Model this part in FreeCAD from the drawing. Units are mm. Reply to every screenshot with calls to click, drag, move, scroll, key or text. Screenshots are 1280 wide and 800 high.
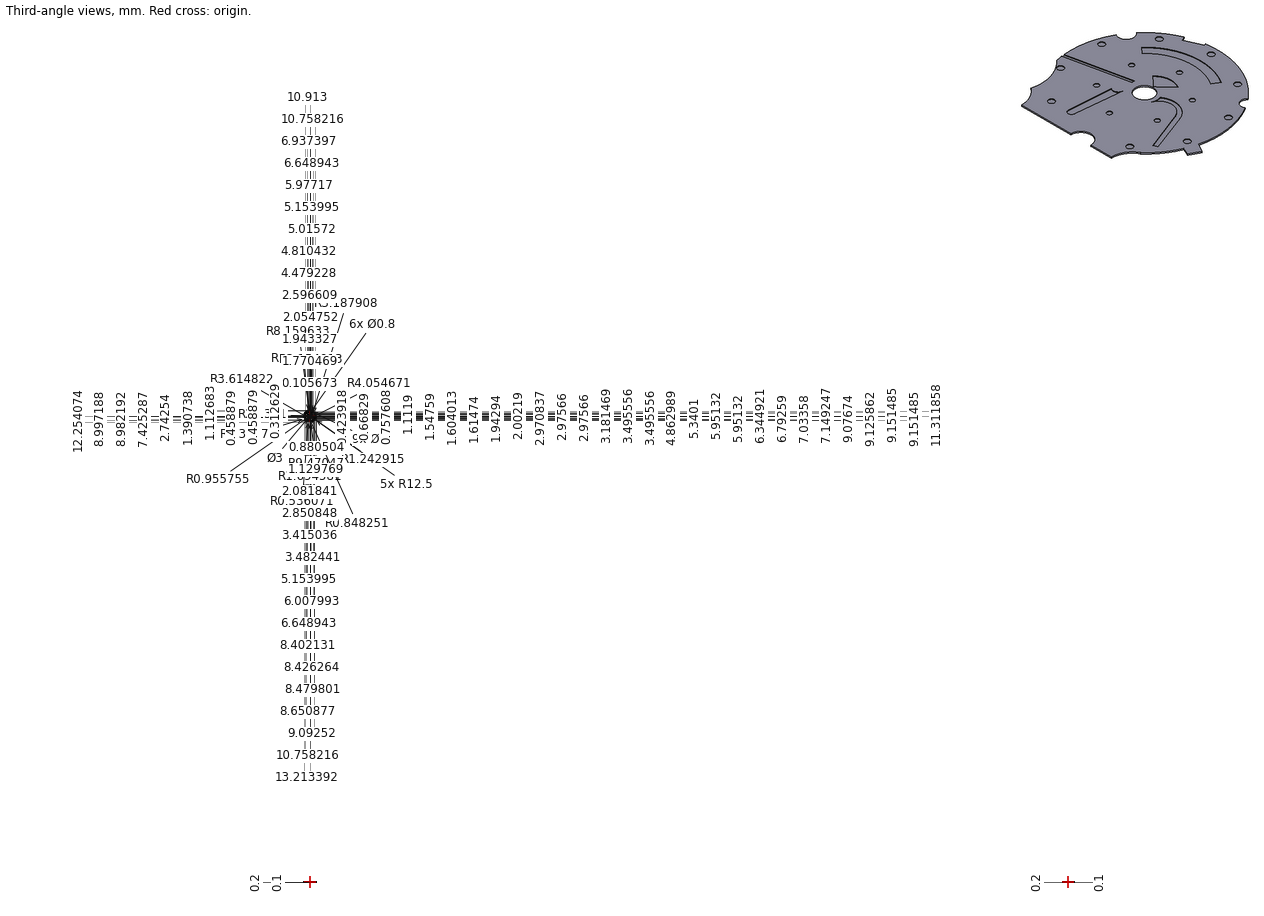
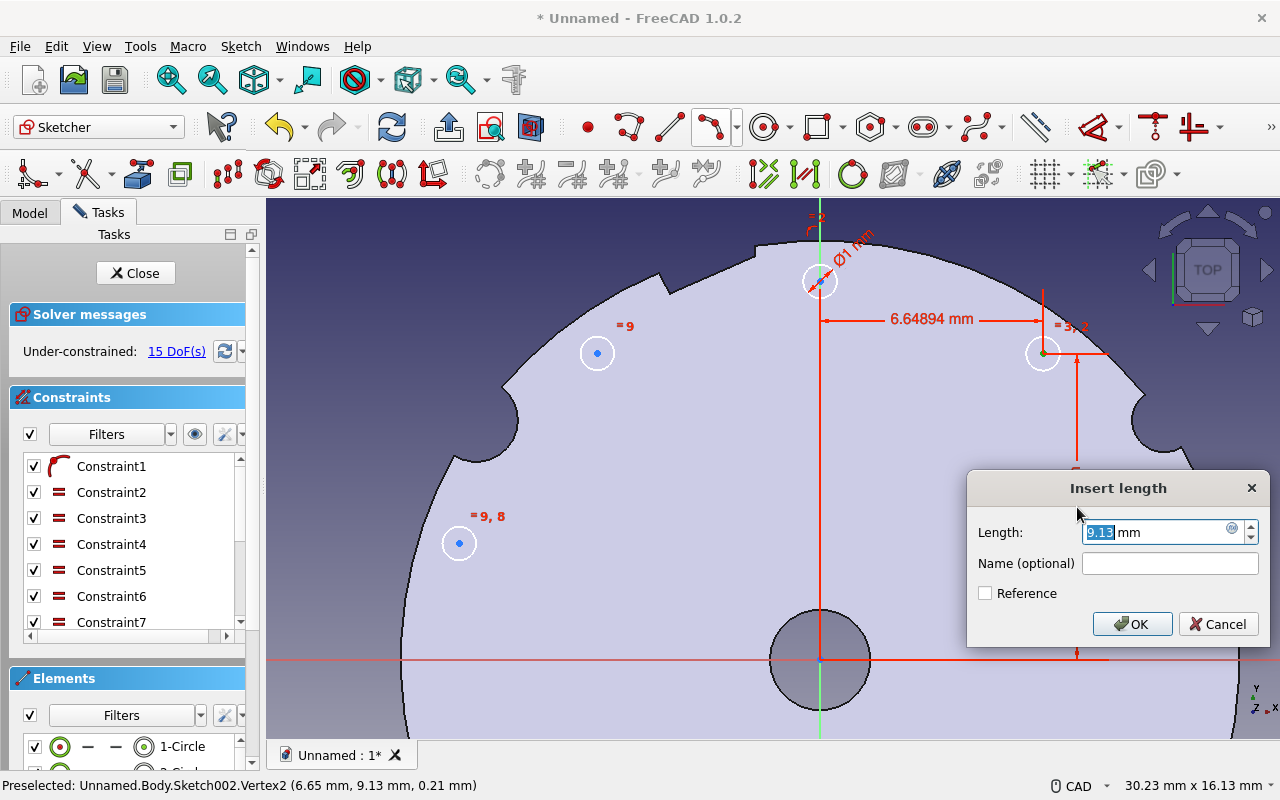
text(9.151485)
key(Return)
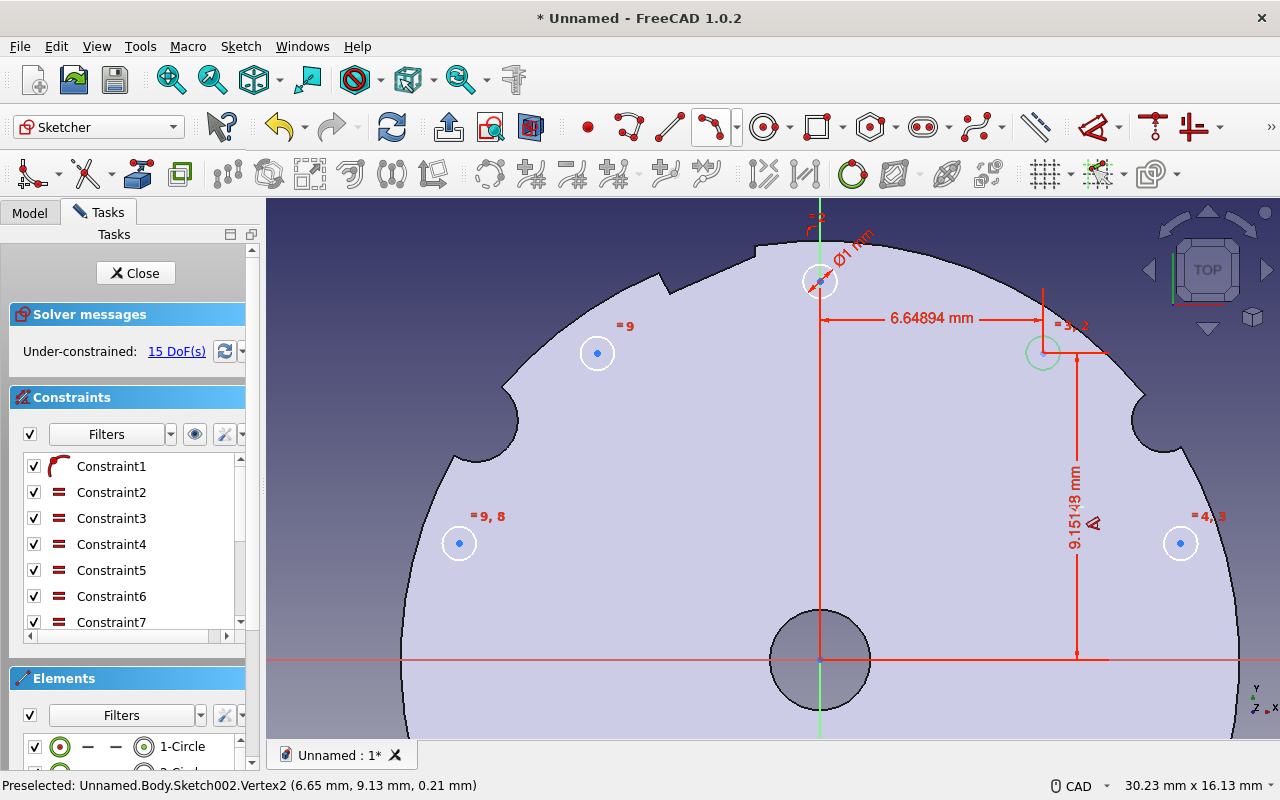
scroll(610, 342, down, 4)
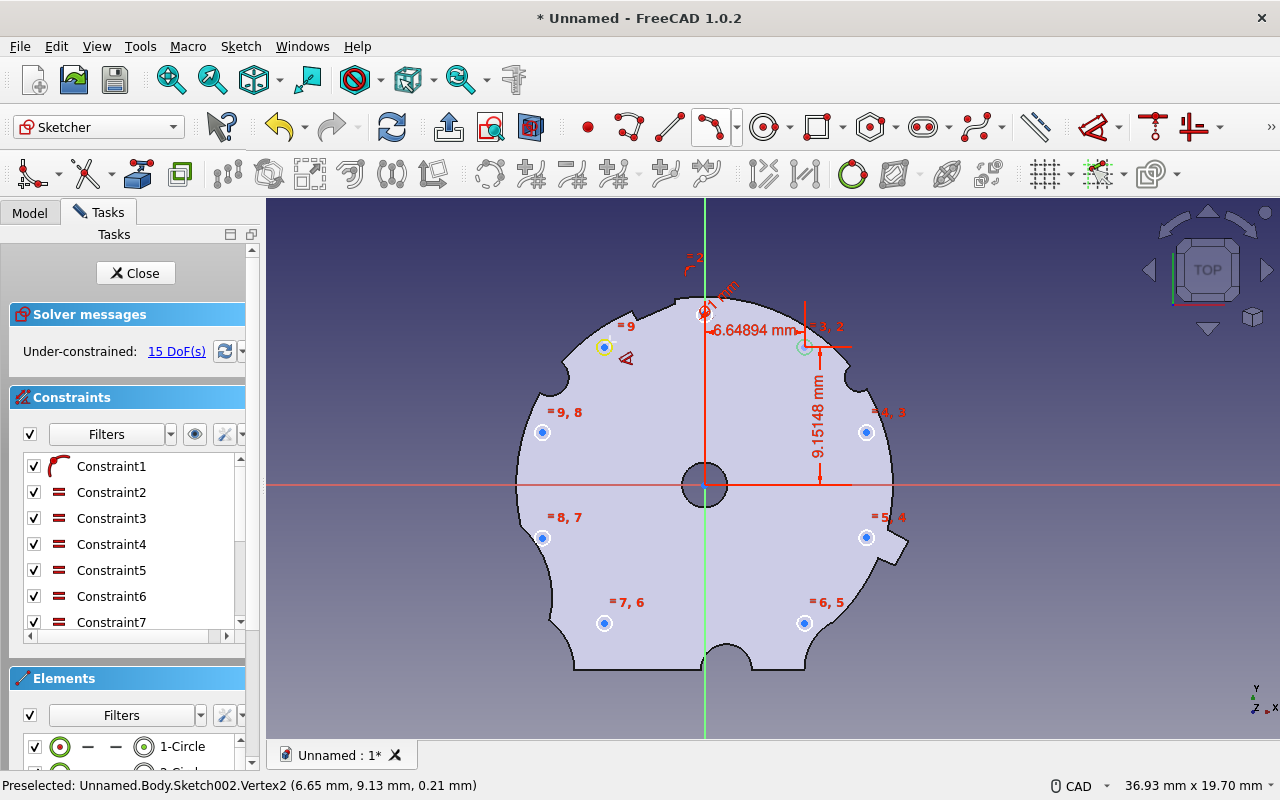
click(867, 433)
click(901, 459)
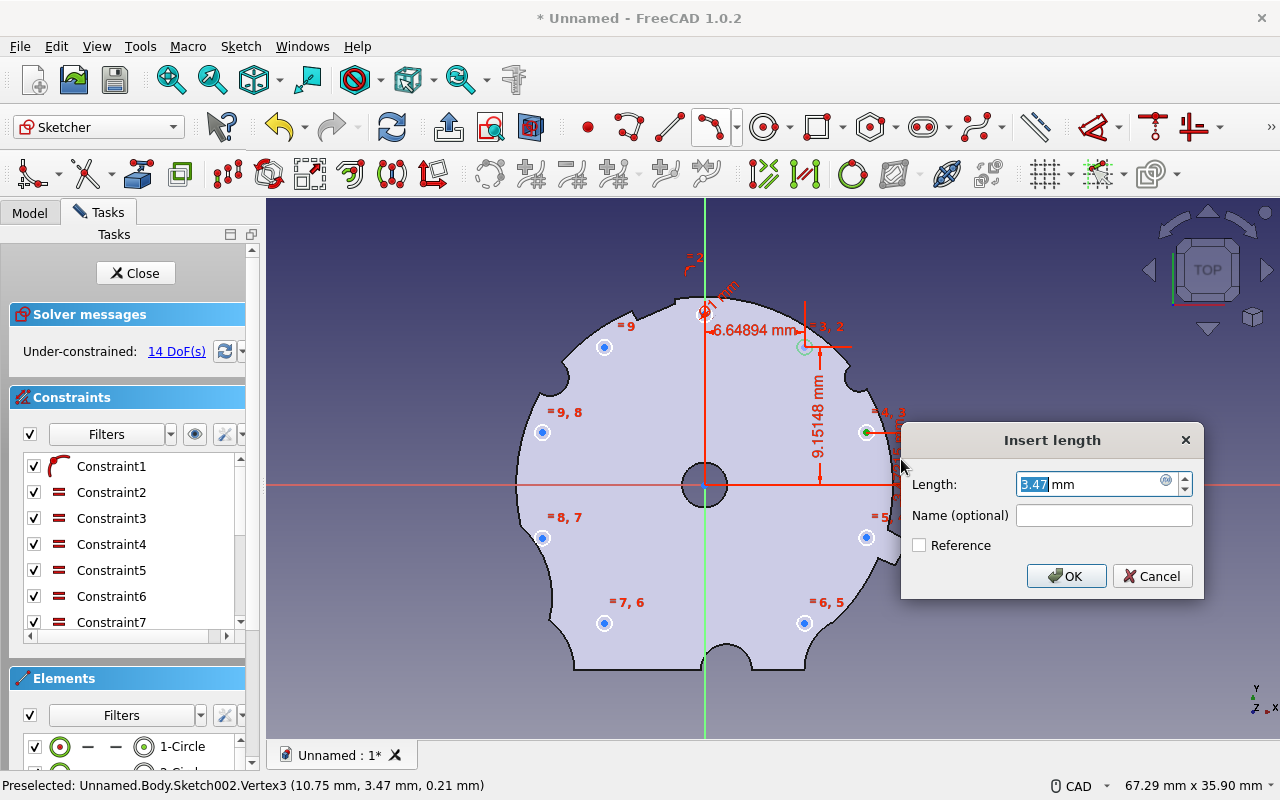
text(3.495556)
key(Return)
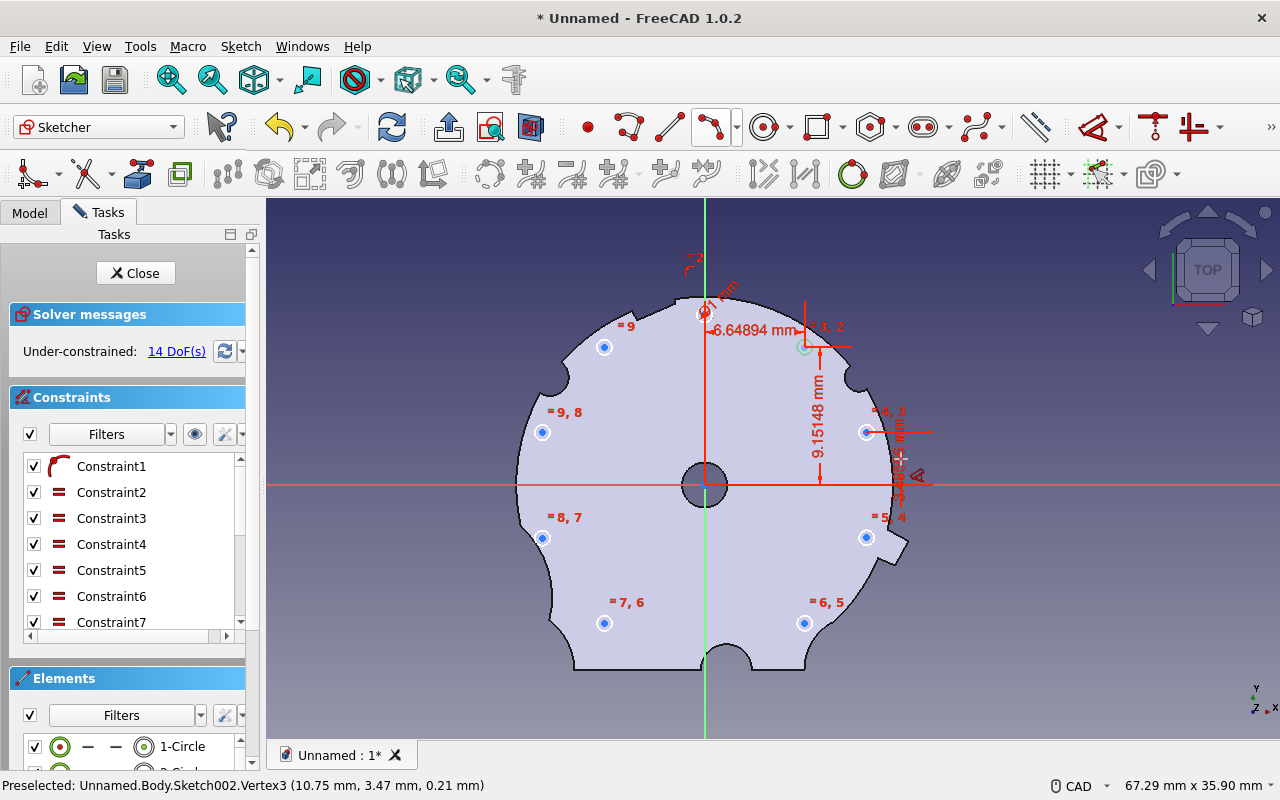
click(867, 538)
click(901, 511)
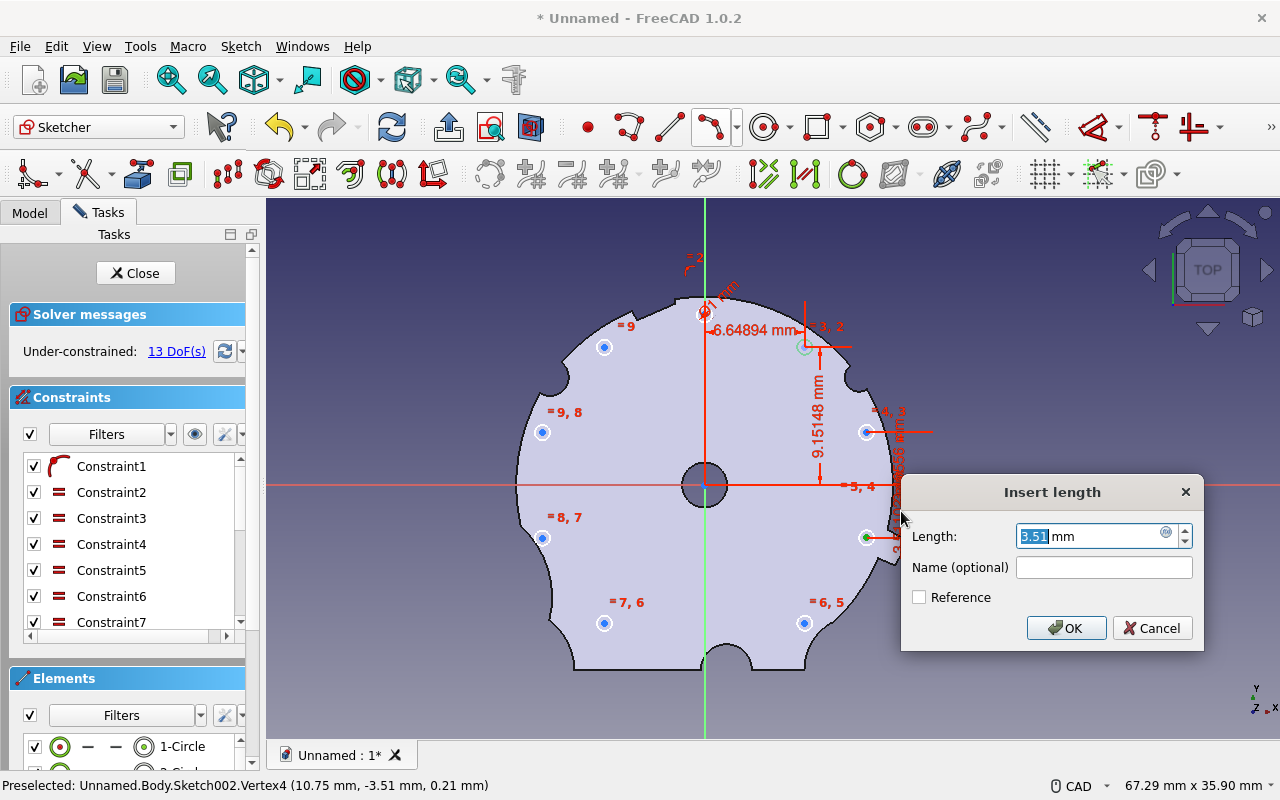
text(3.495556)
key(Return)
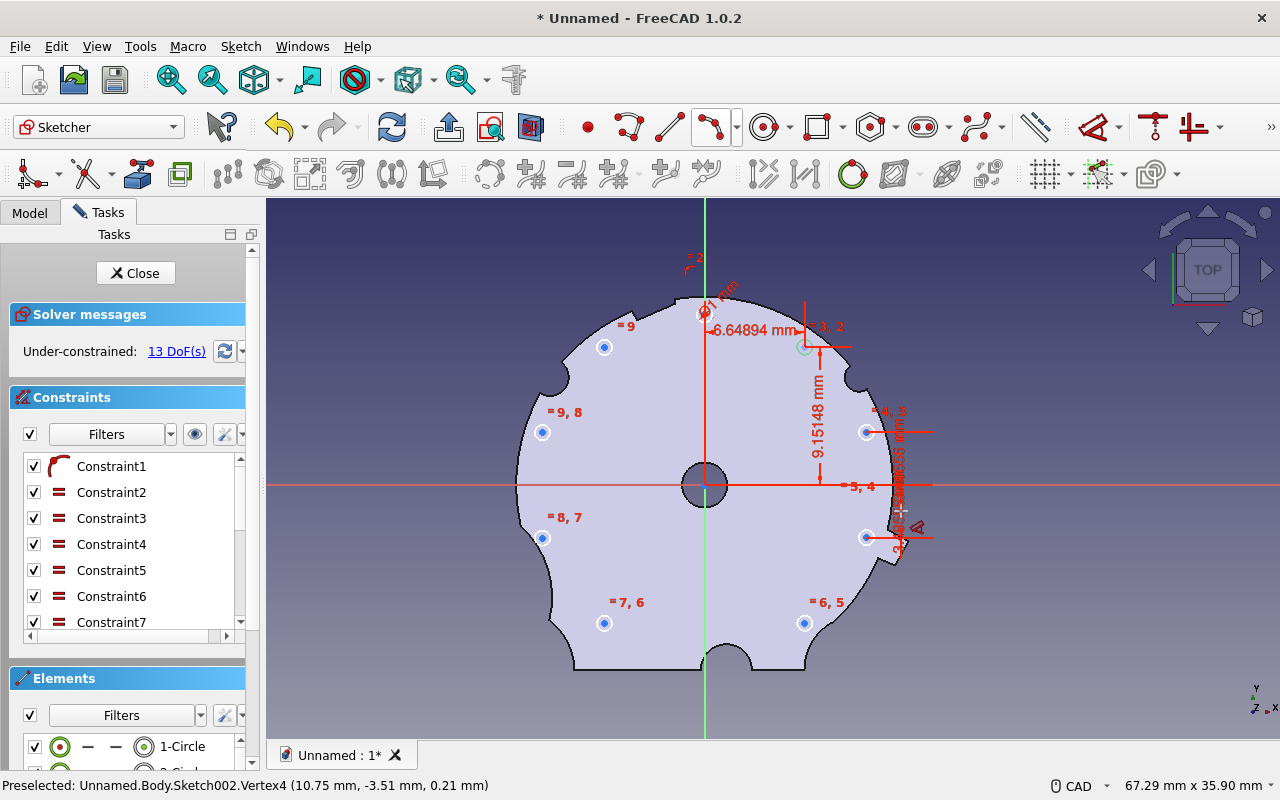
click(805, 623)
click(755, 657)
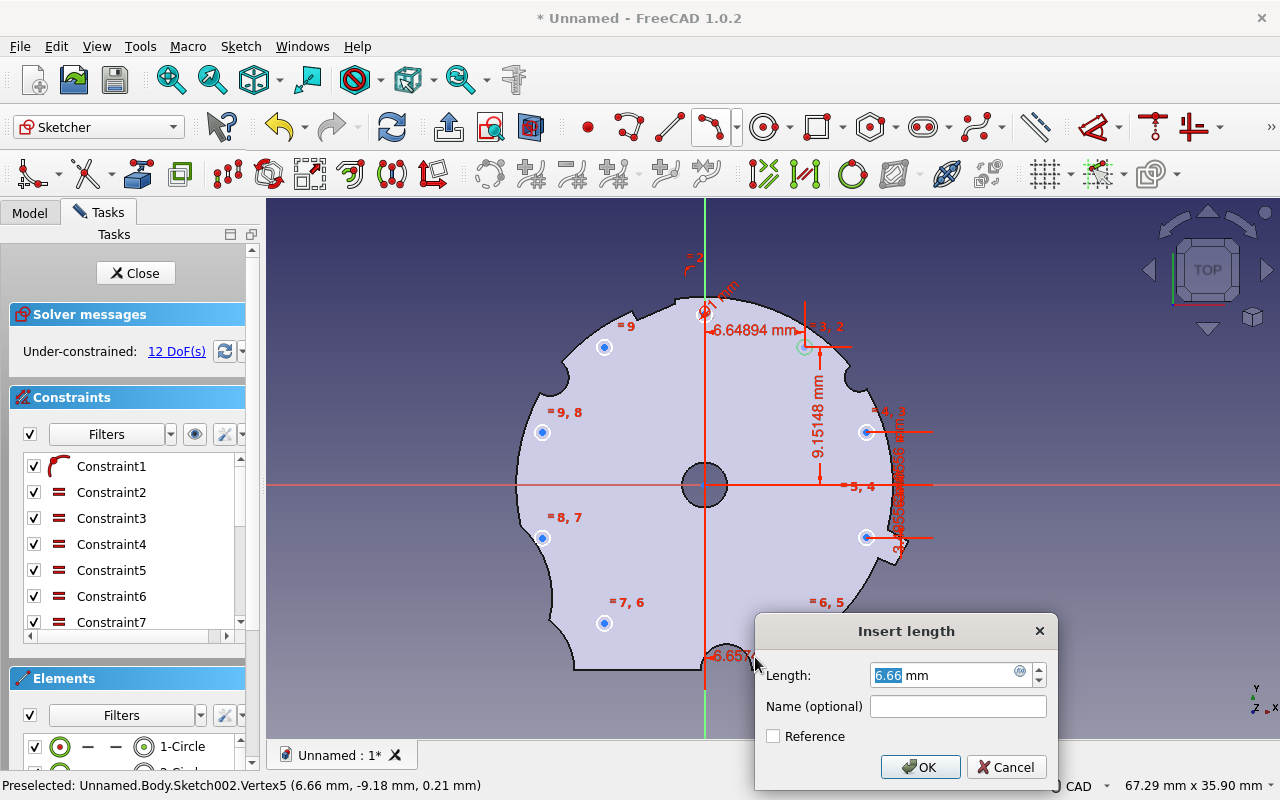
text(6.648943)
key(Return)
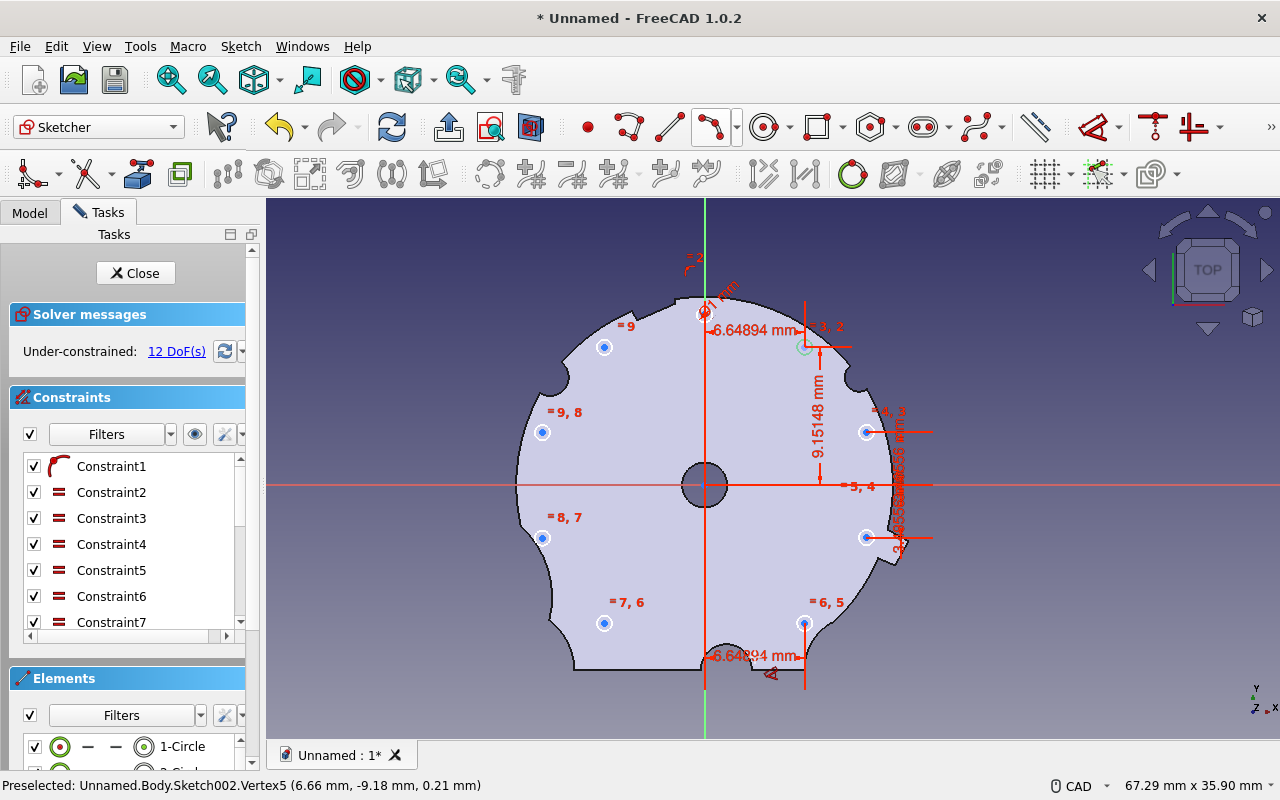
click(805, 623)
click(839, 554)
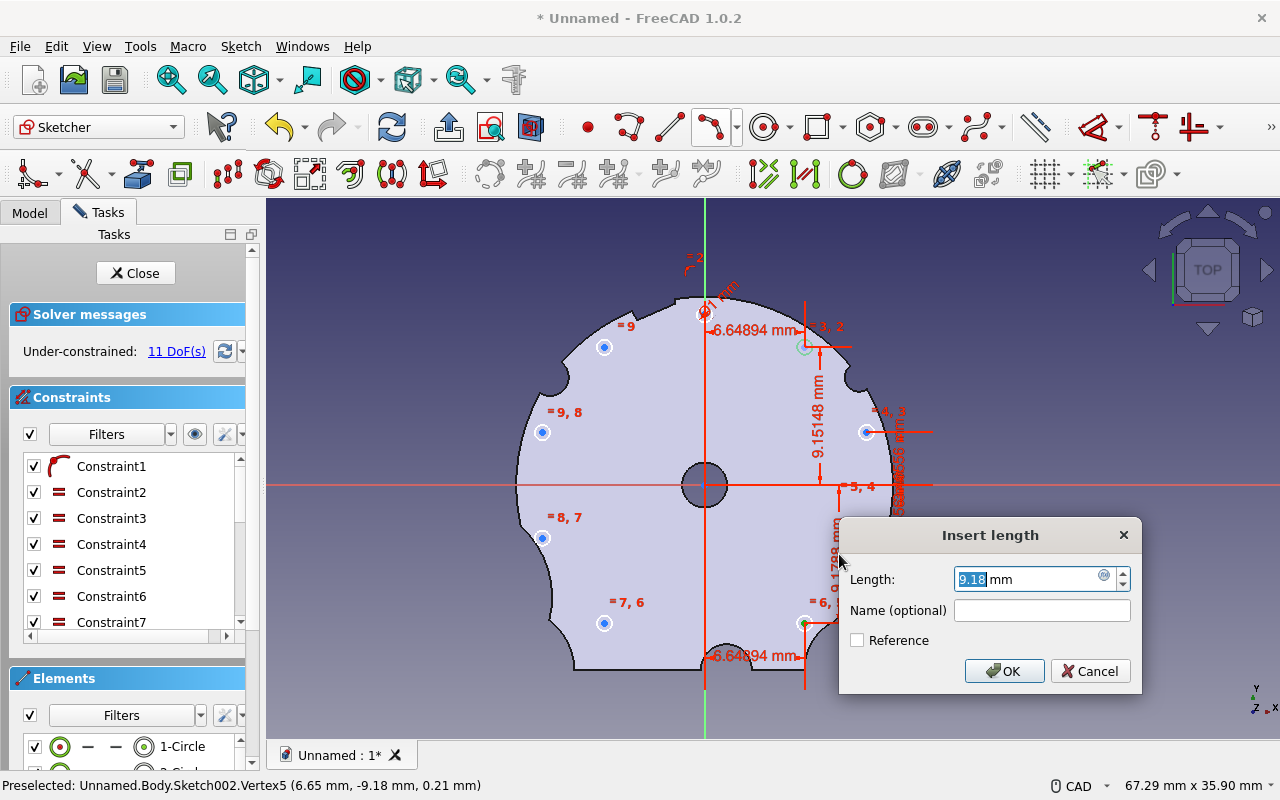
text(9.151485)
key(Return)